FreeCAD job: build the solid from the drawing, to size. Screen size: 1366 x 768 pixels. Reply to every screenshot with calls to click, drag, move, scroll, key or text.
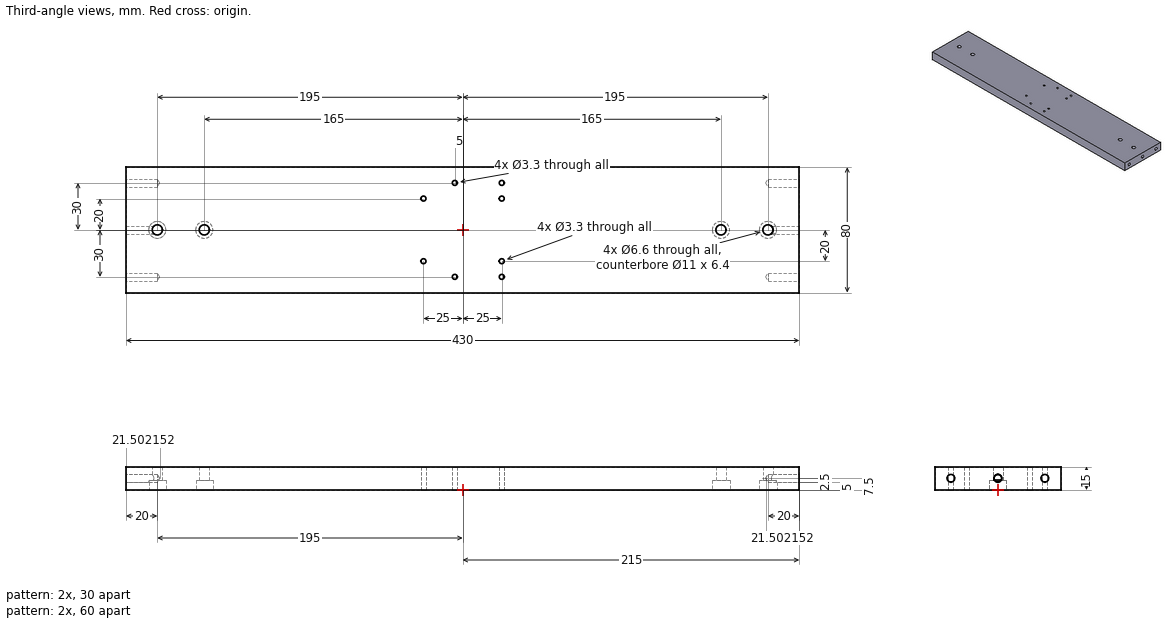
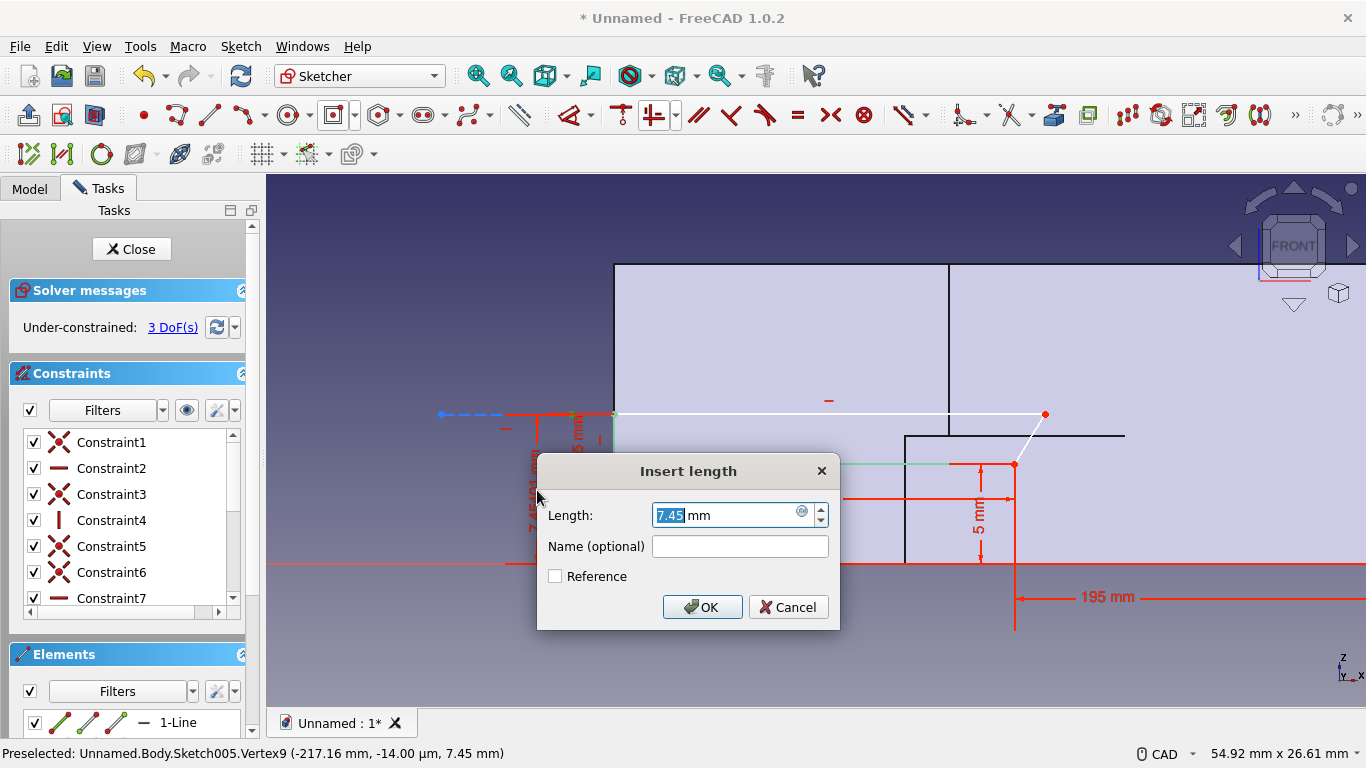
text(7.5)
key(Return)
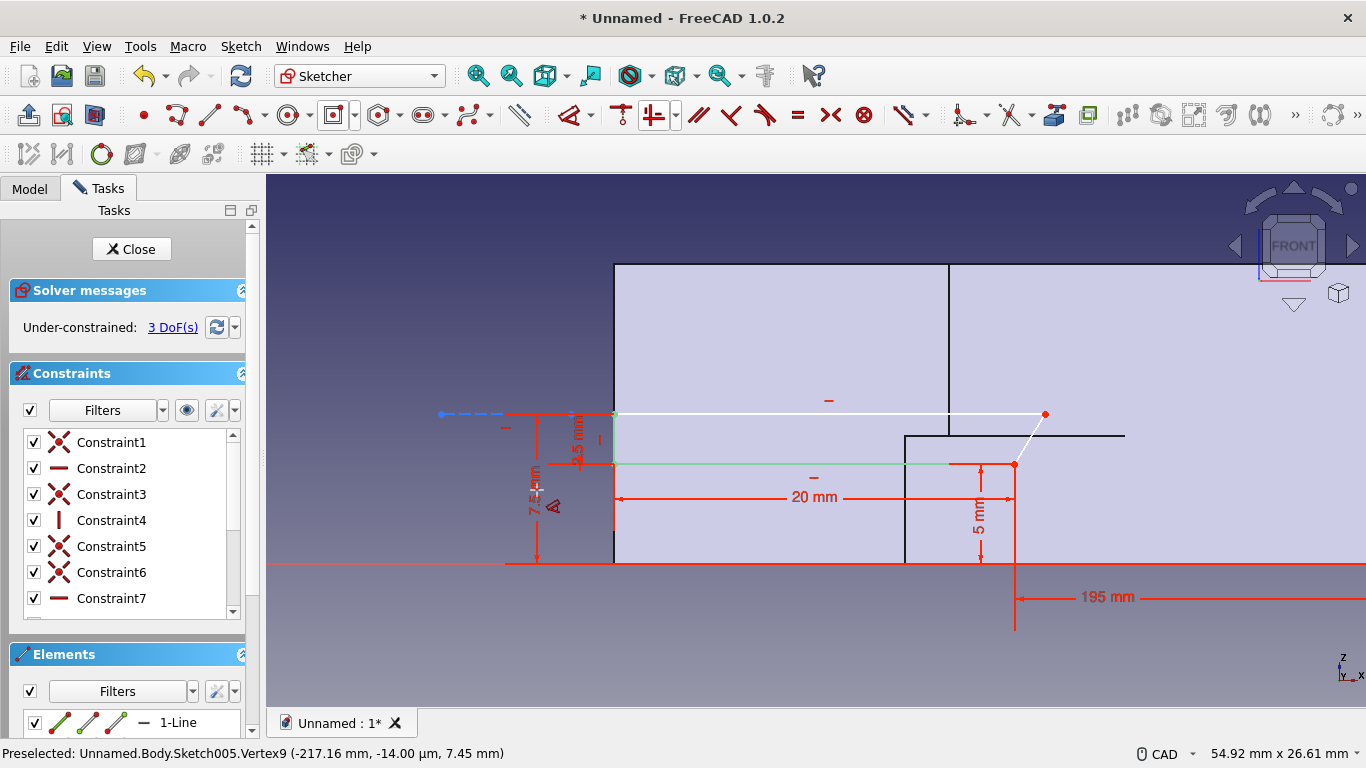
click(743, 414)
click(830, 380)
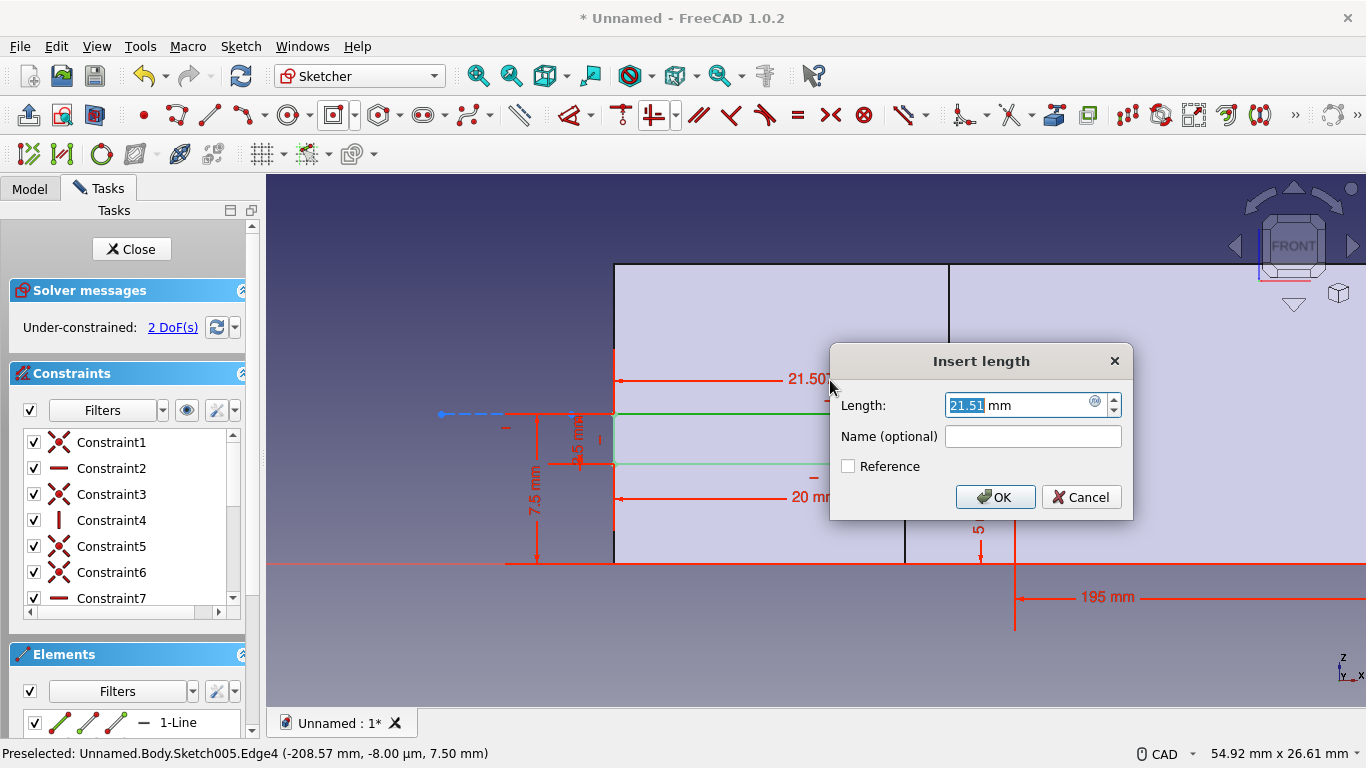
text(21.502152)
key(Return)
key(Escape)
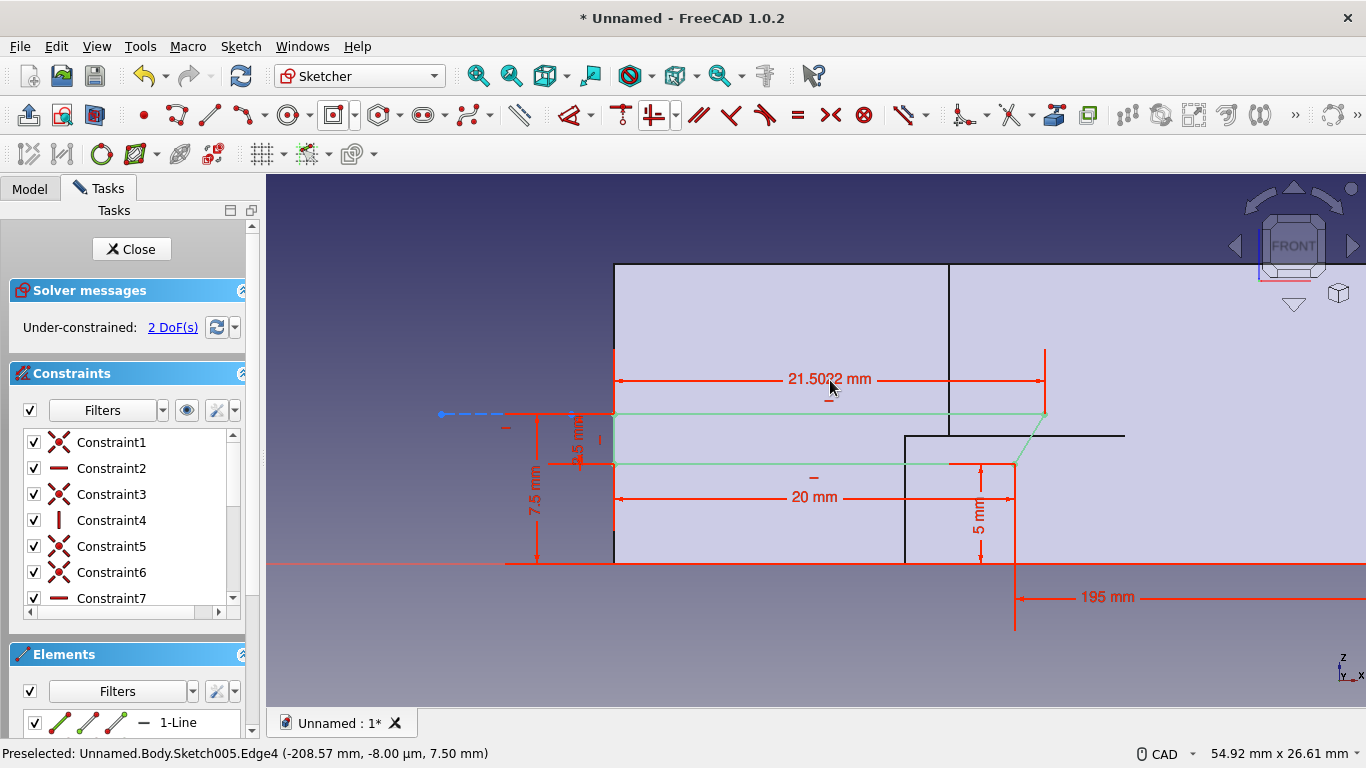
click(132, 249)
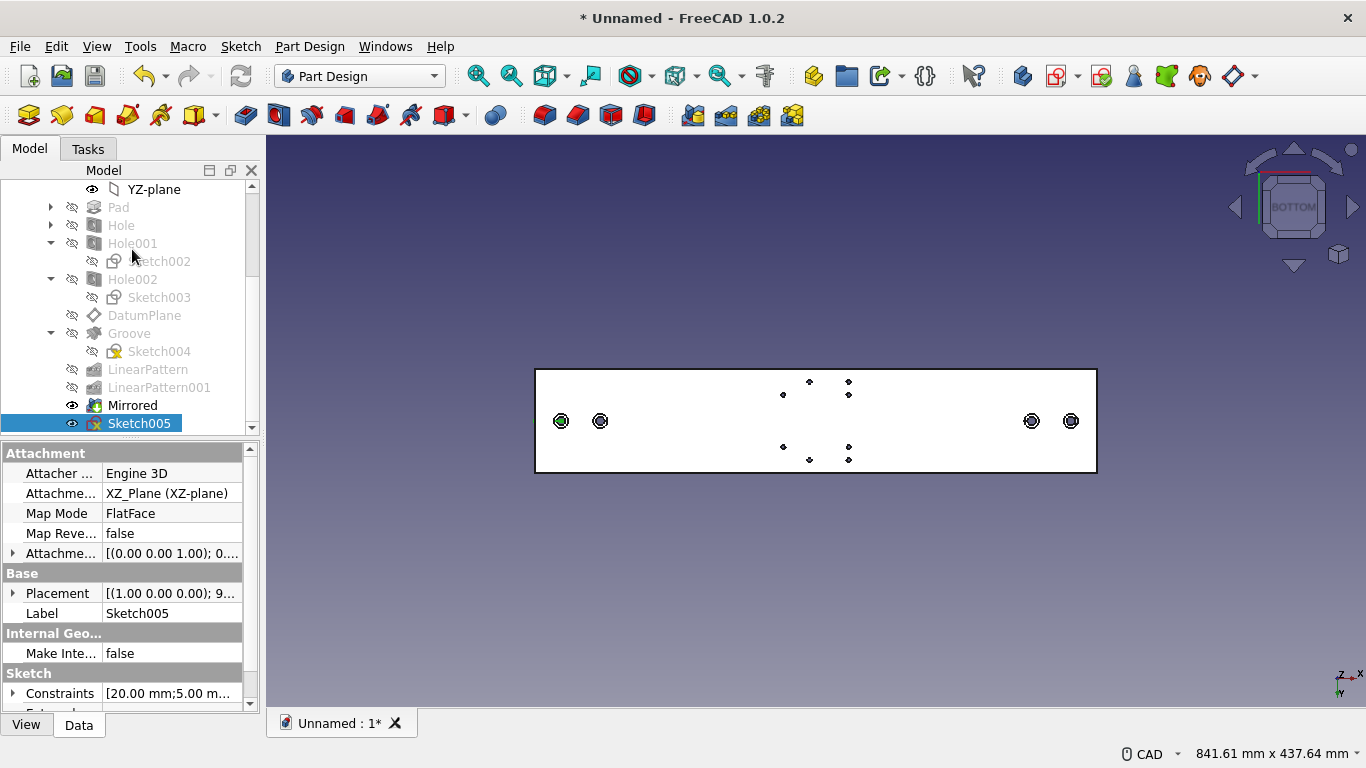
click(312, 116)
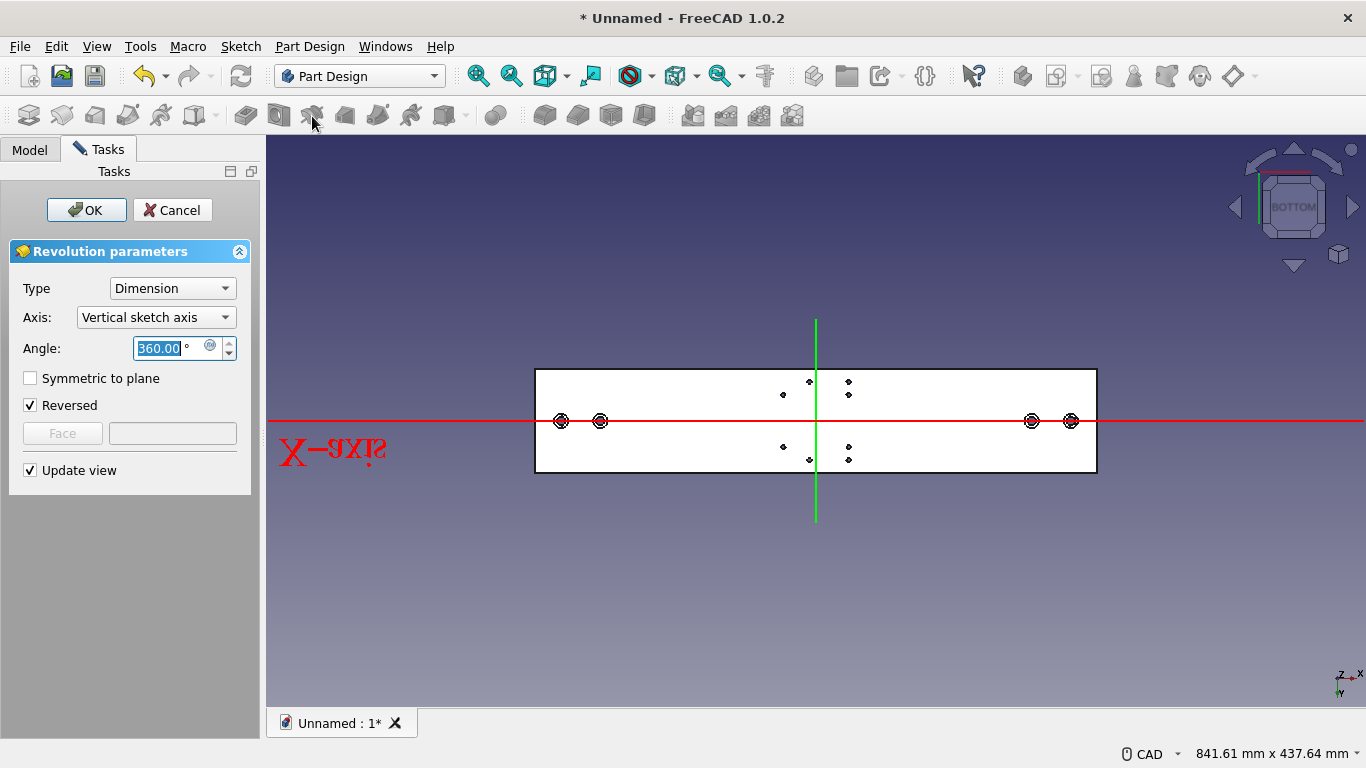
click(157, 318)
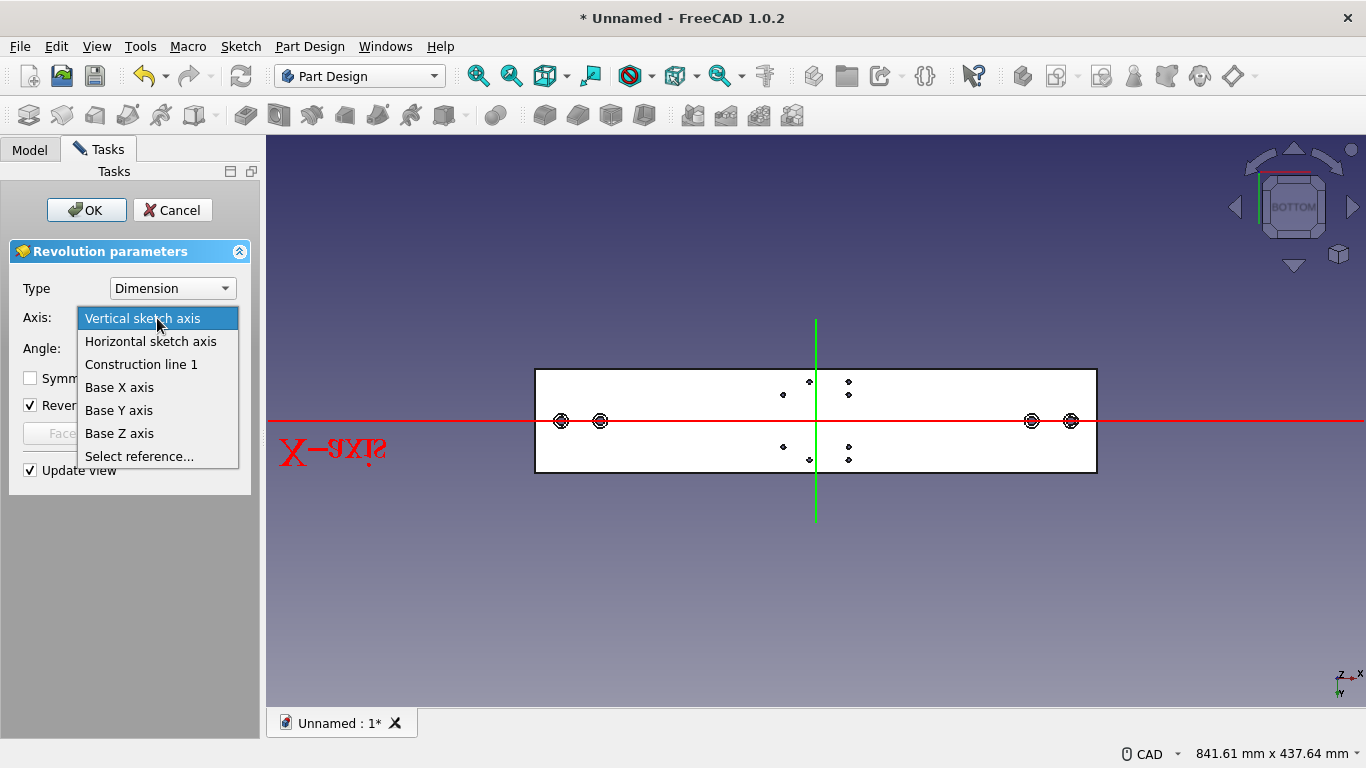
click(156, 364)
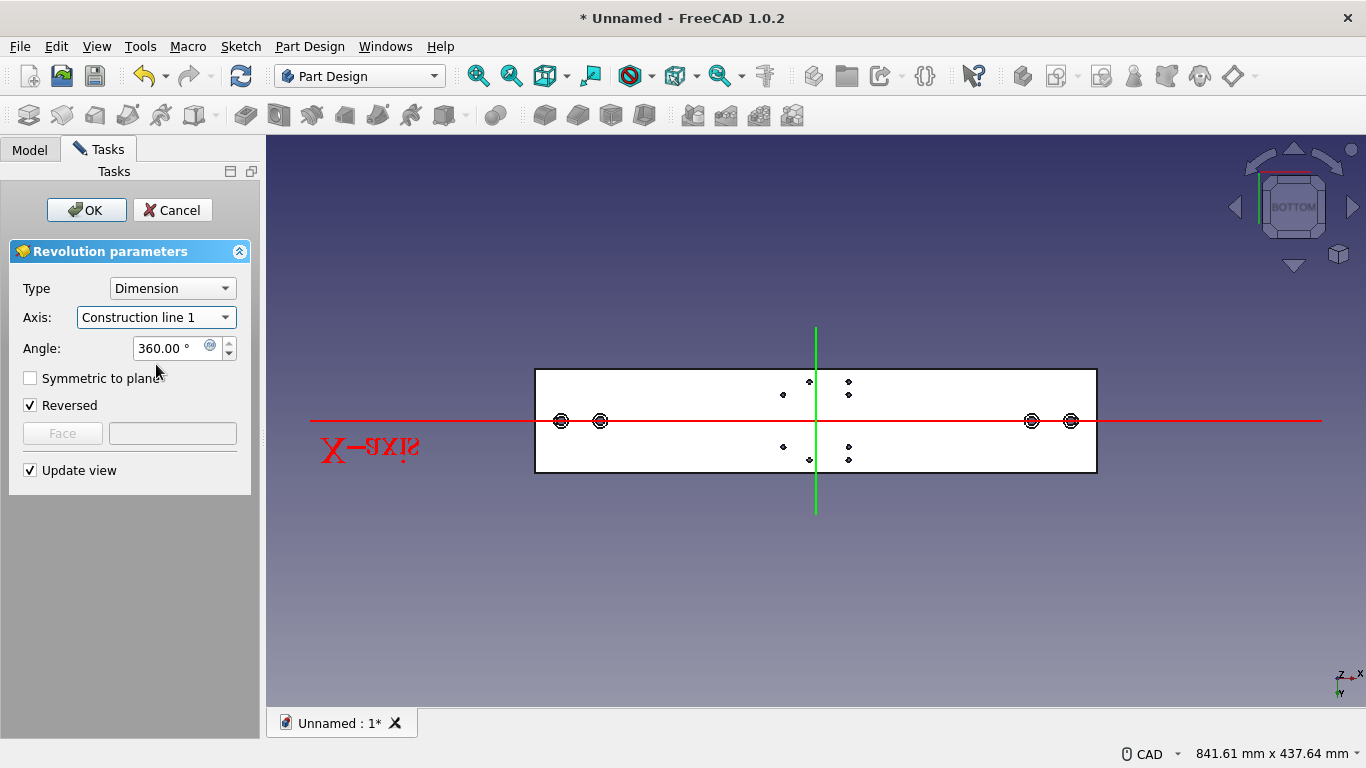
click(87, 210)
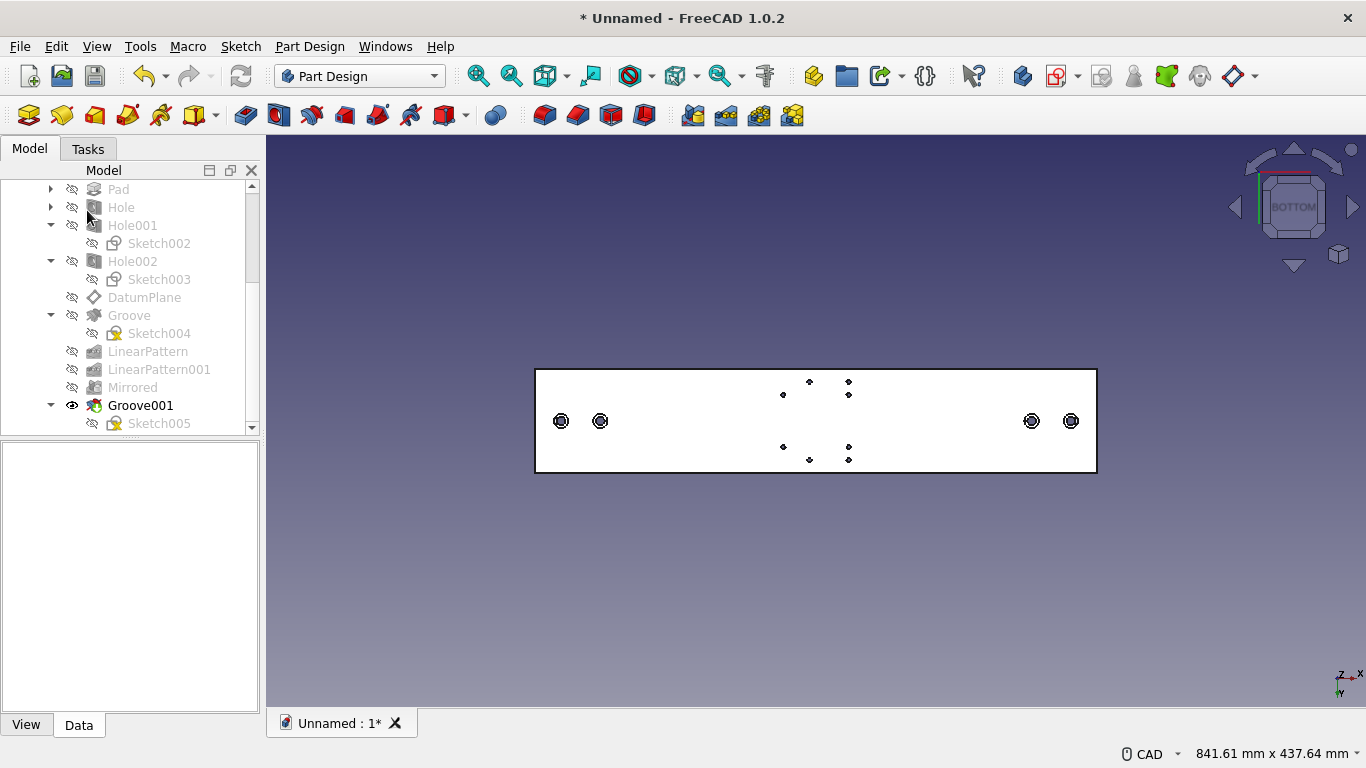
scroll(141, 311, down, 3)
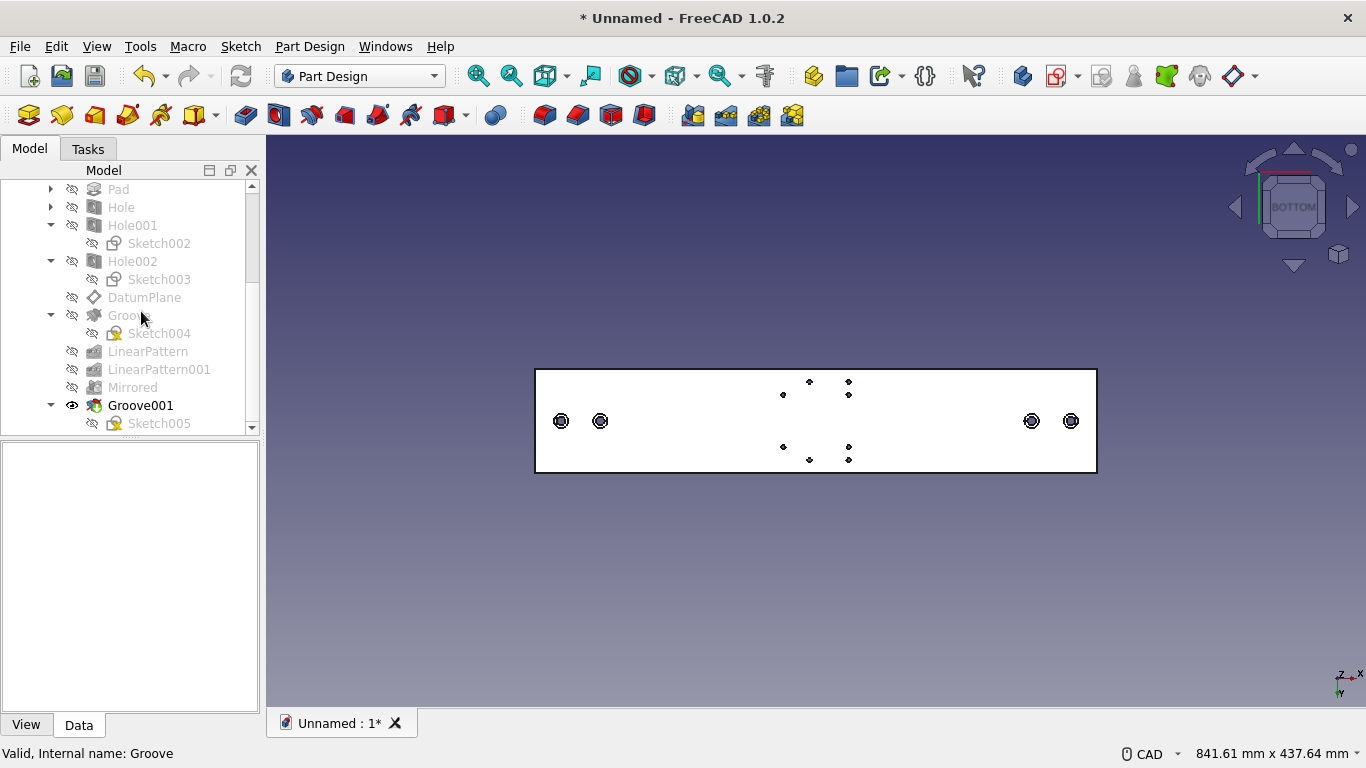
scroll(141, 311, up, 15)